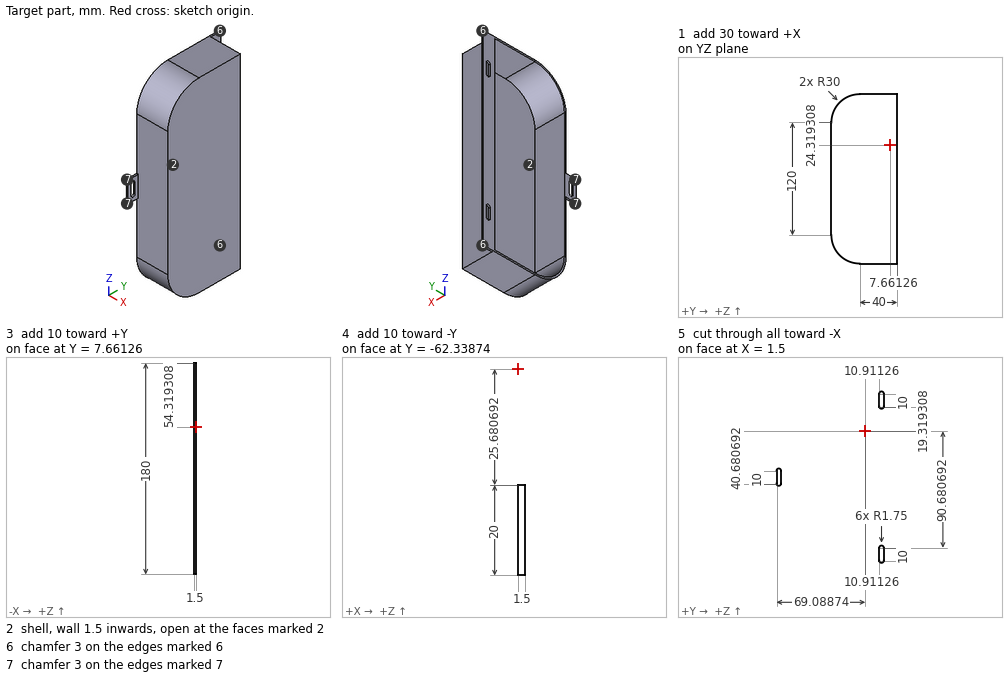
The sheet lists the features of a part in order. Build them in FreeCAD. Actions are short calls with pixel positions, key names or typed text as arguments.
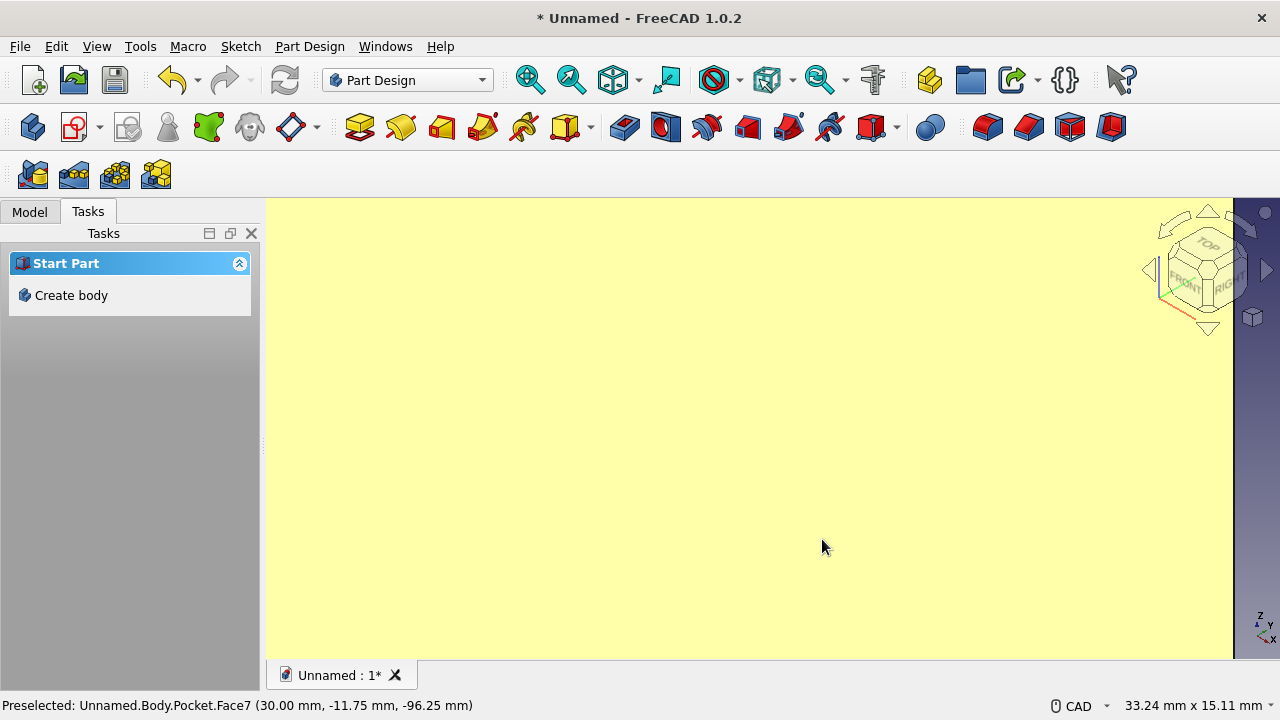
click(531, 80)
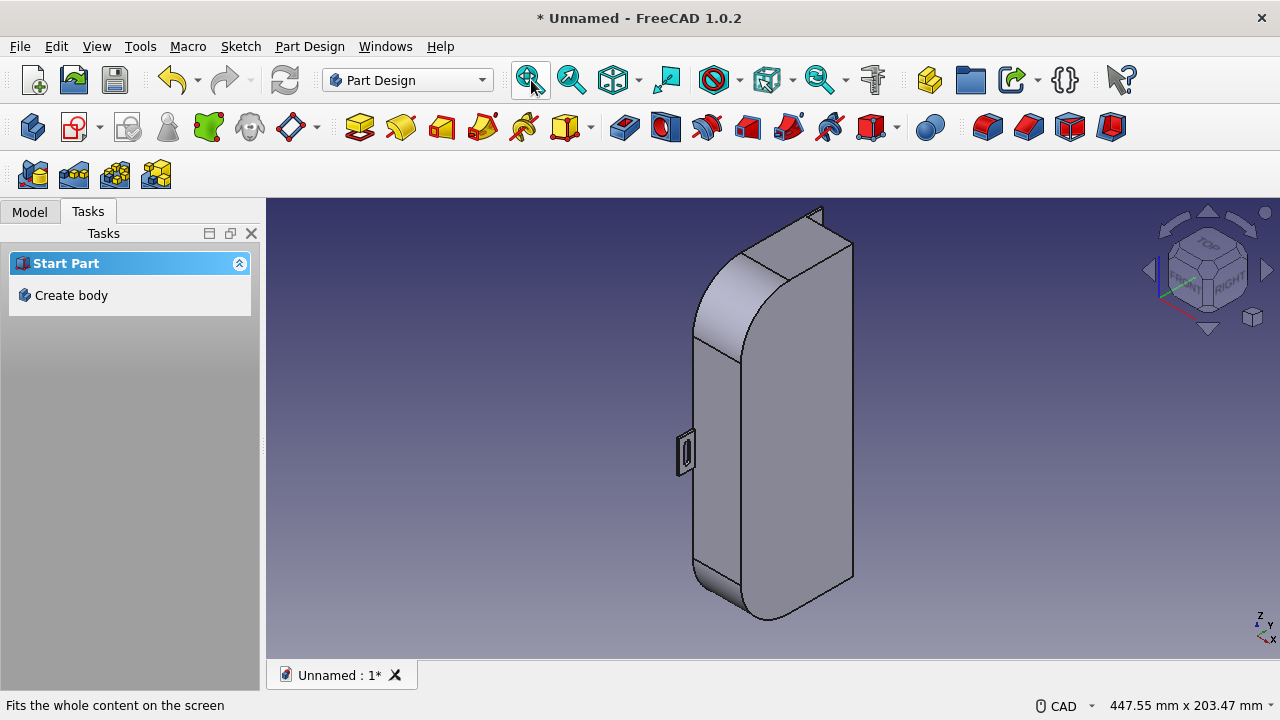
key(2)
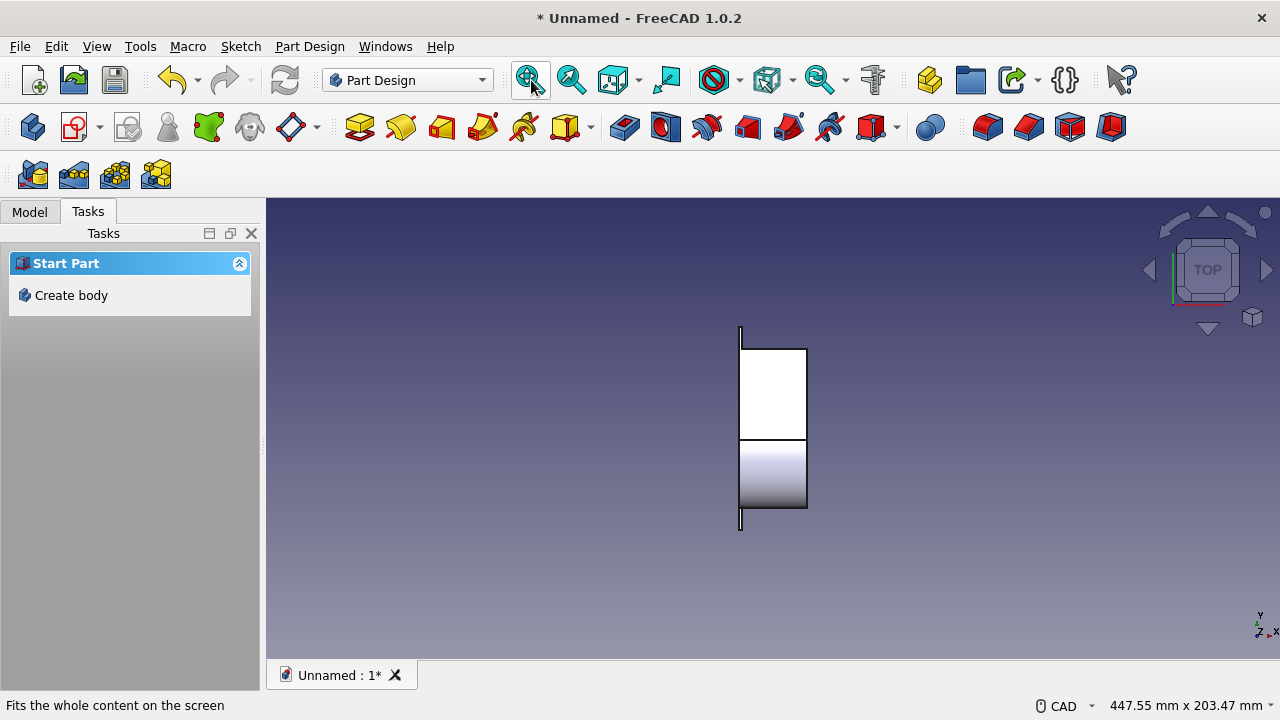
click(531, 80)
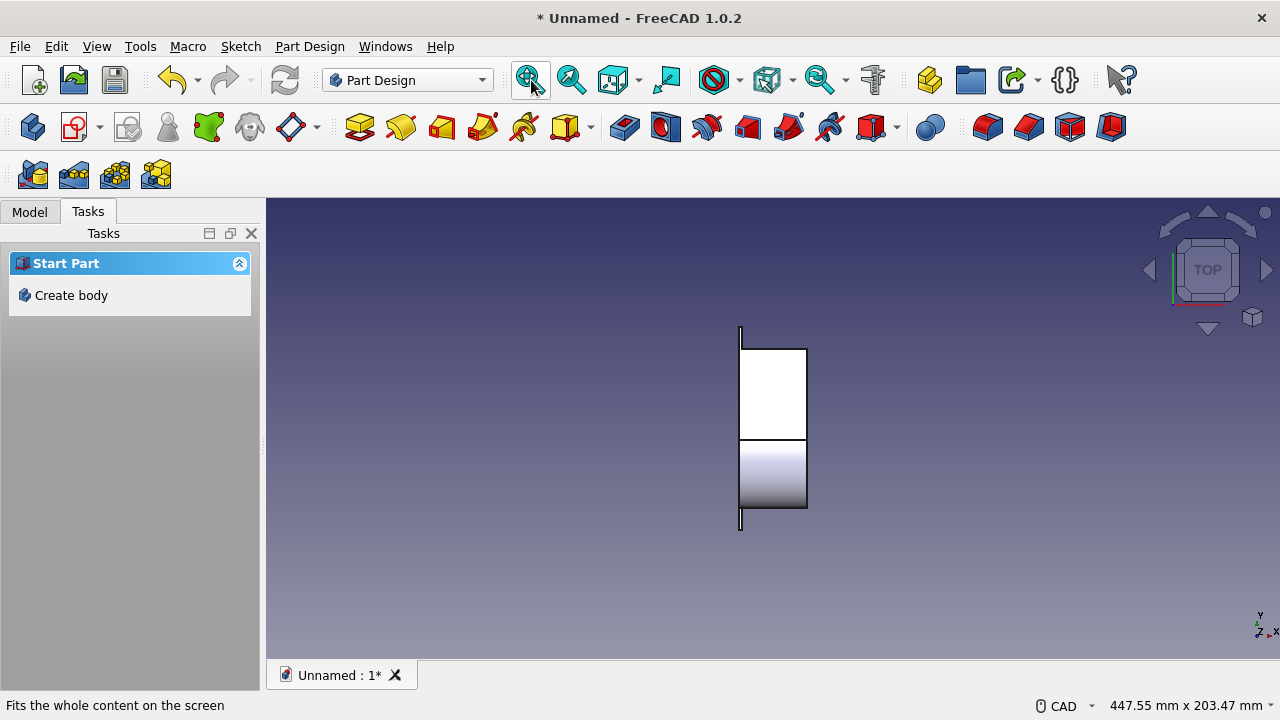
scroll(741, 326, up, 13)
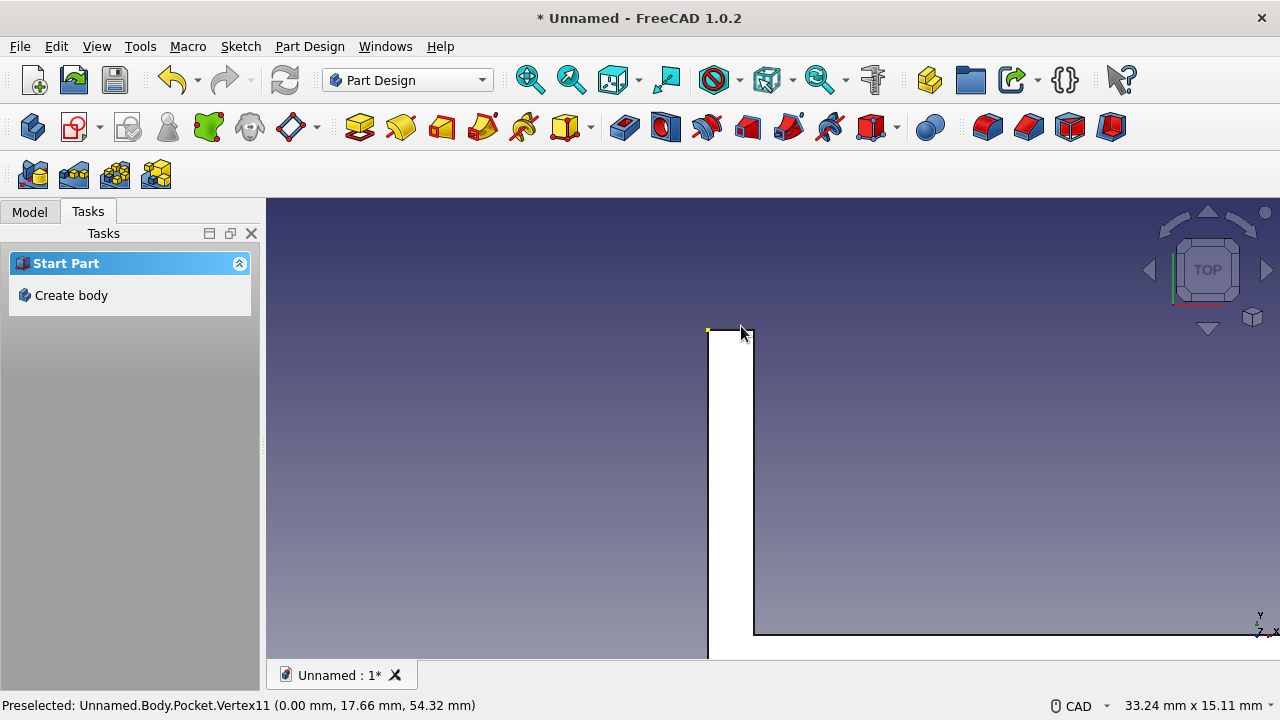
click(731, 329)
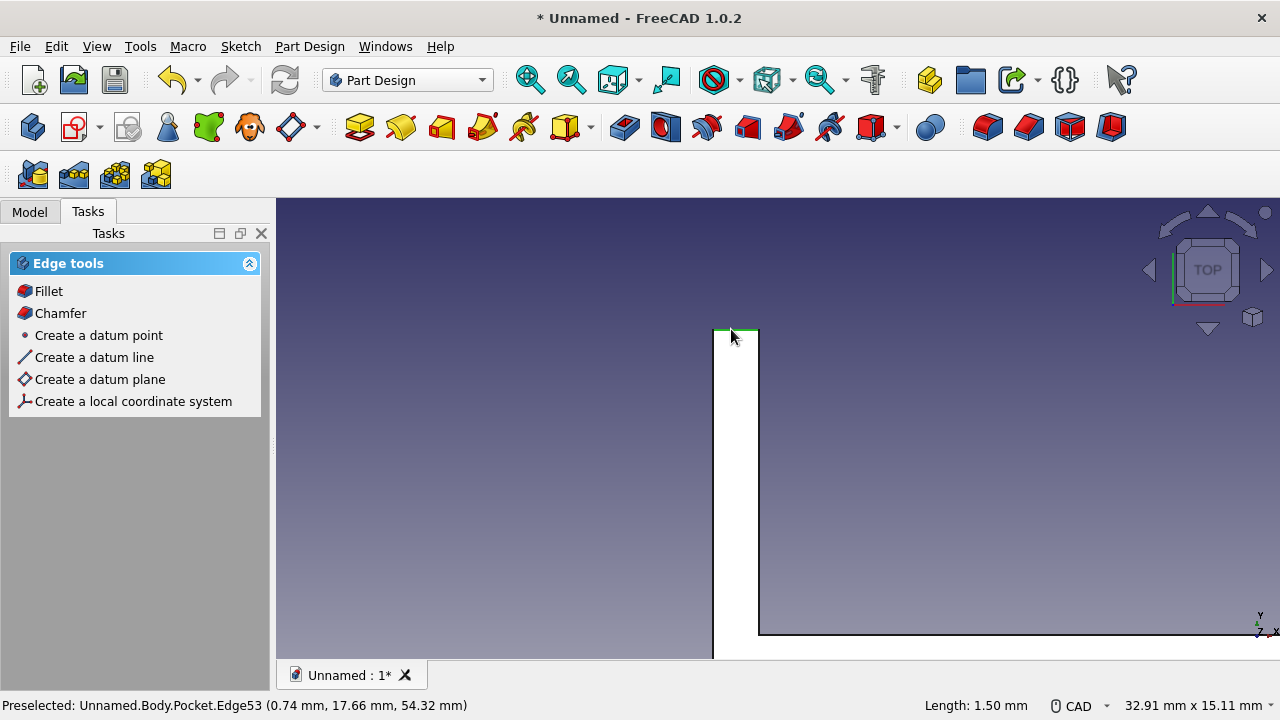
click(531, 80)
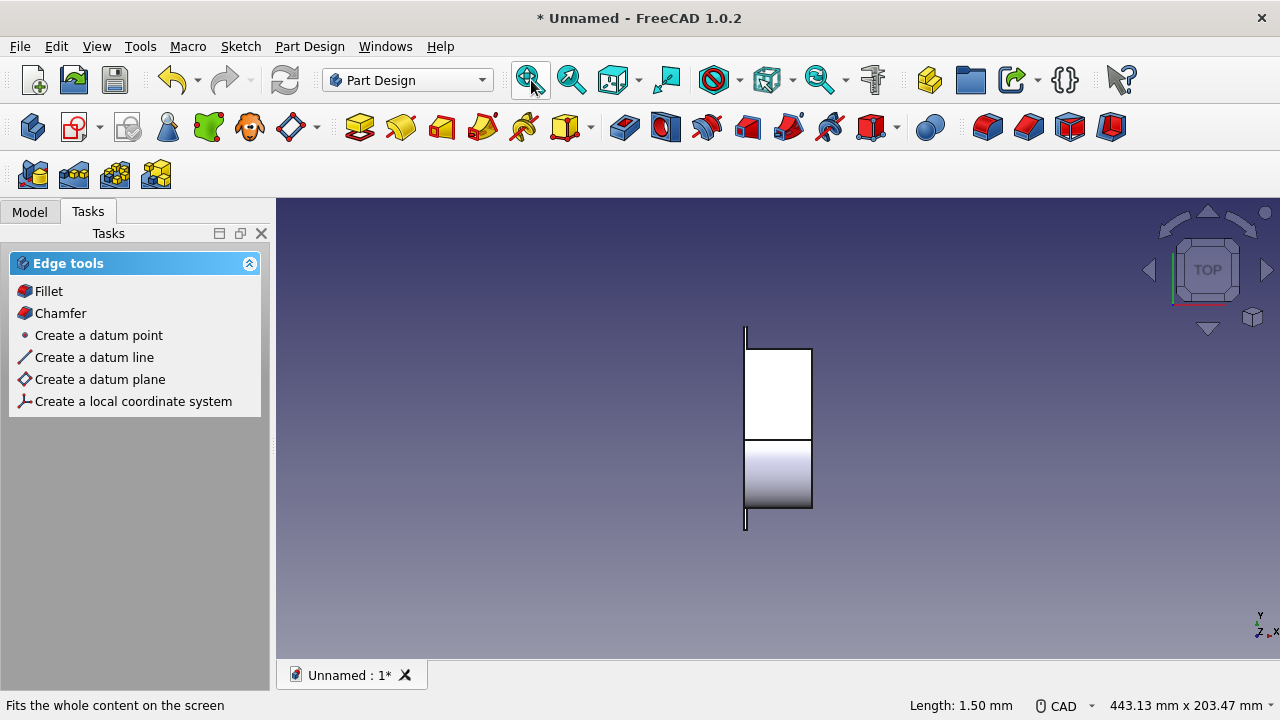
key(1)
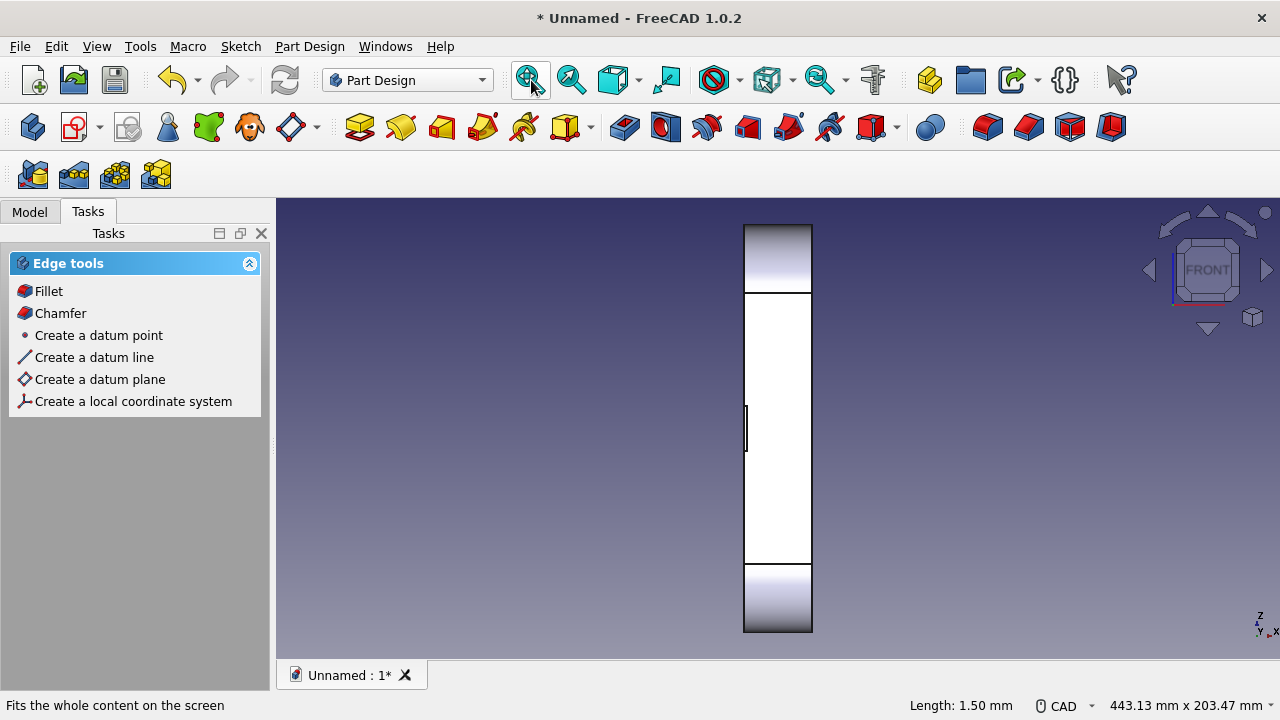
key(3)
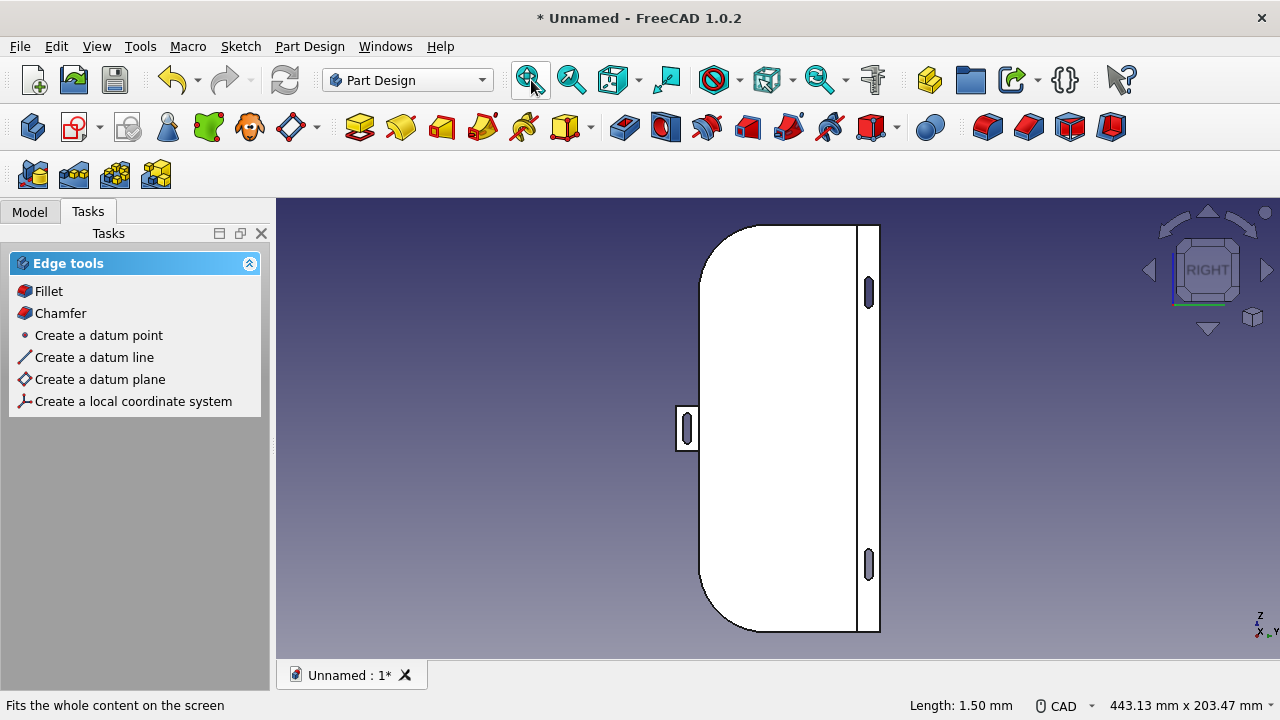
key(5)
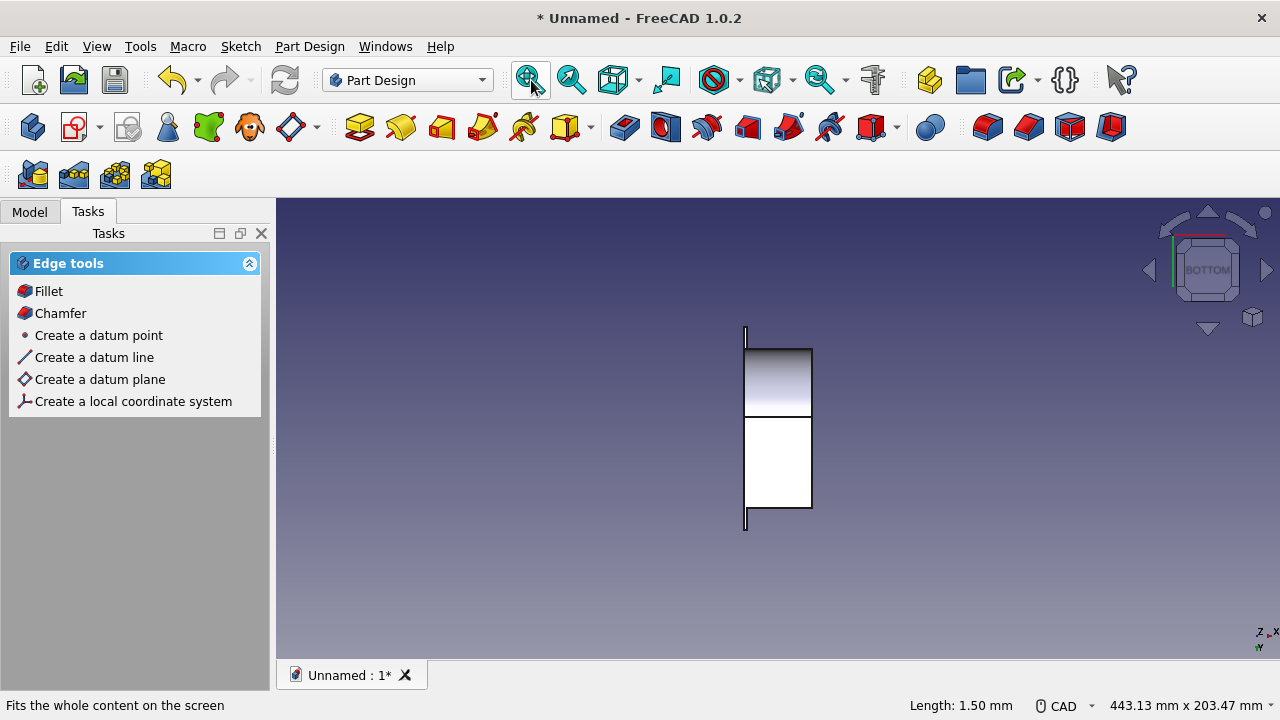
click(531, 80)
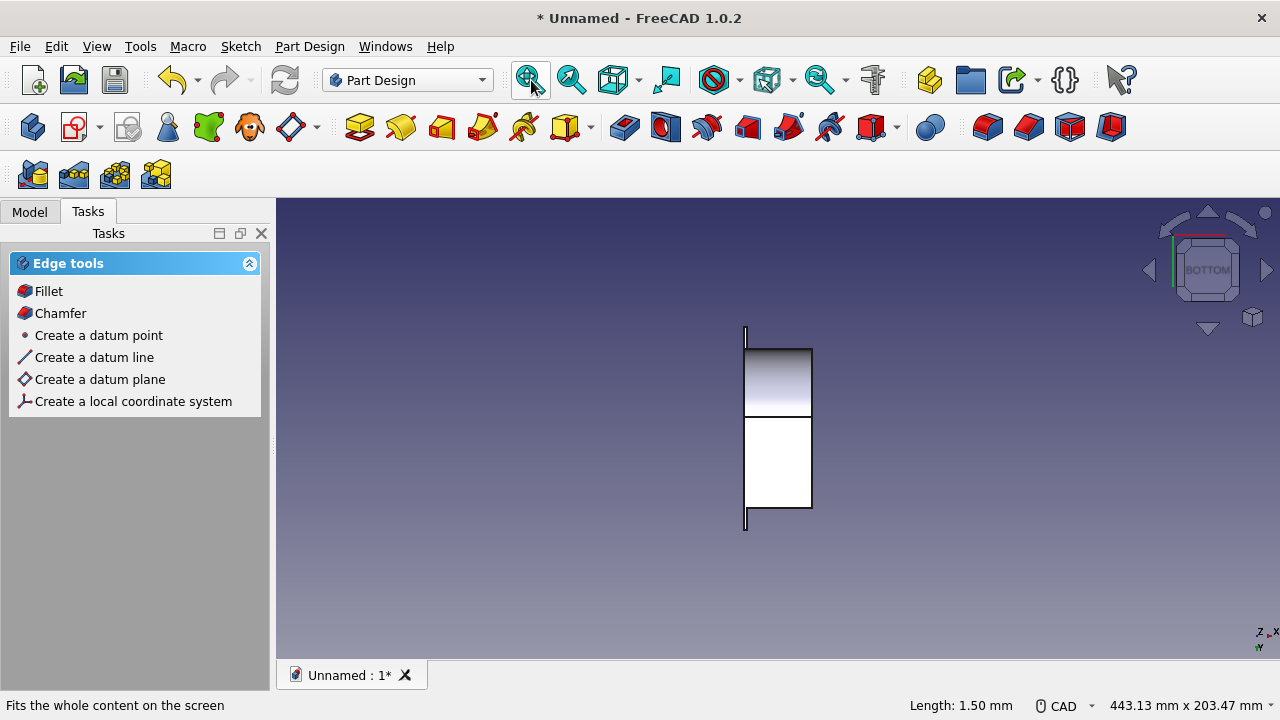
scroll(746, 529, up, 13)